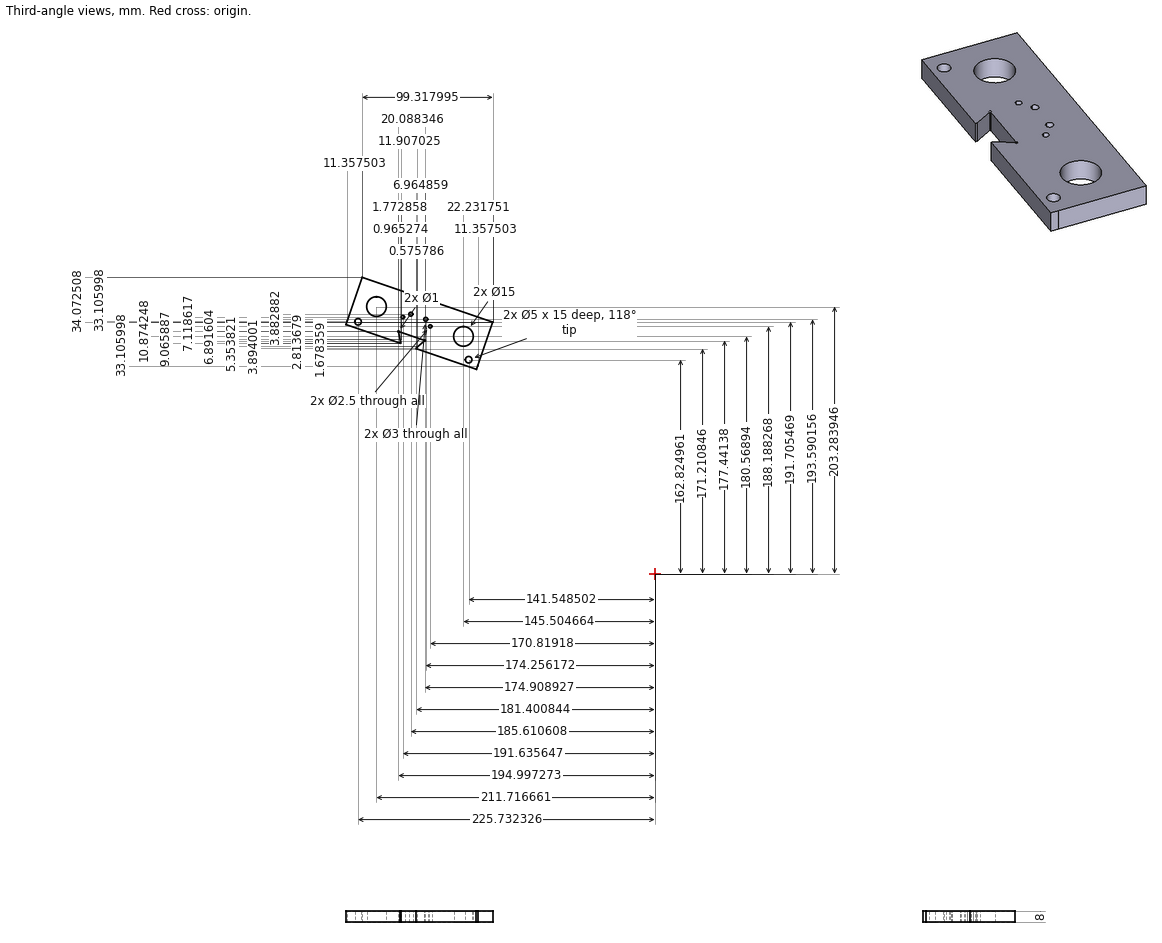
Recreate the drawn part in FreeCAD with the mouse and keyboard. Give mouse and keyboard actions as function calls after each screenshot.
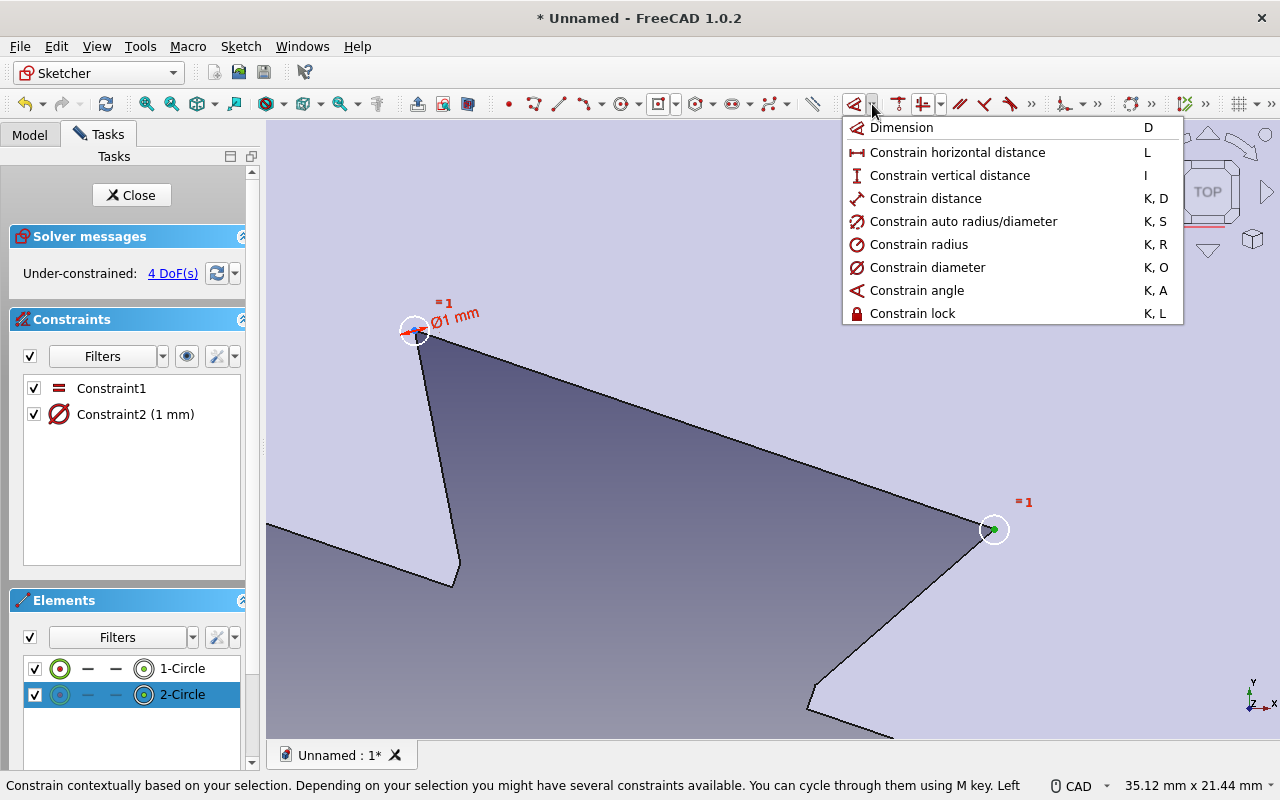
click(1013, 176)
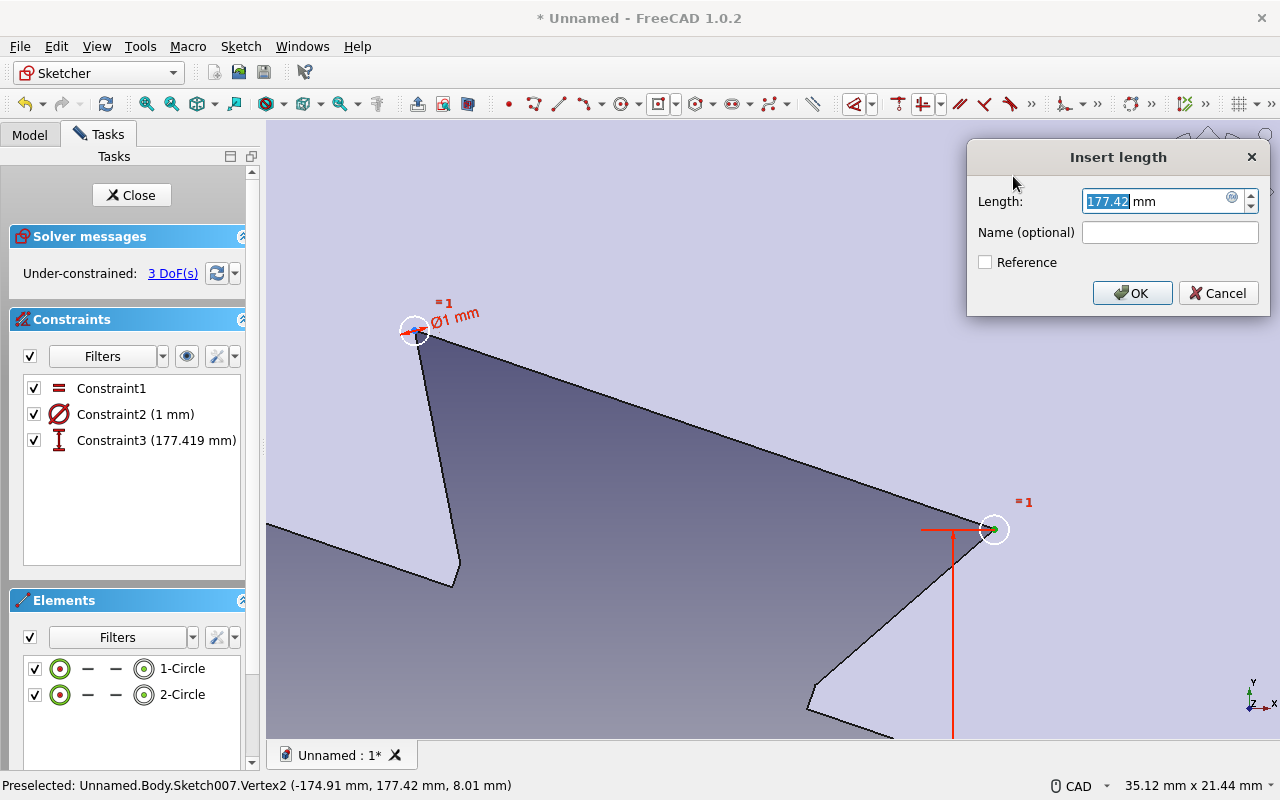
text(177.44138)
key(Return)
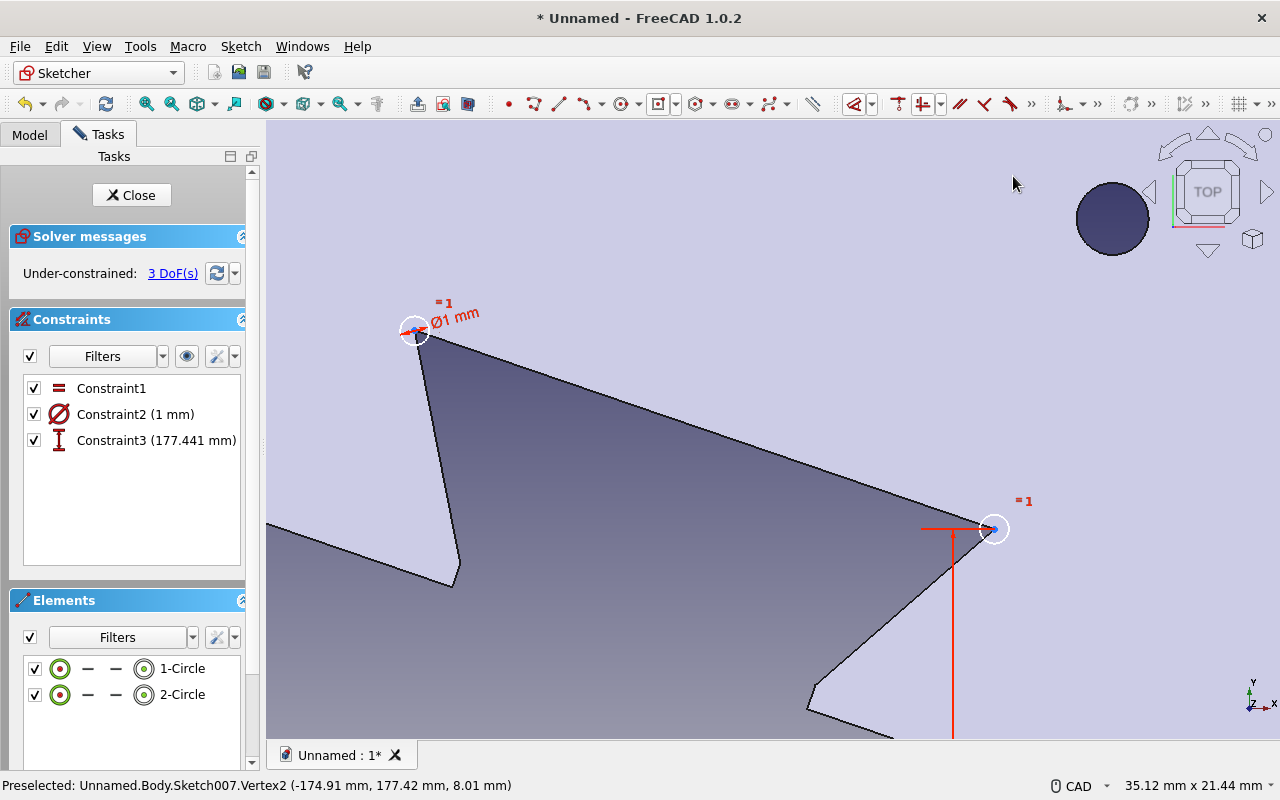
click(415, 331)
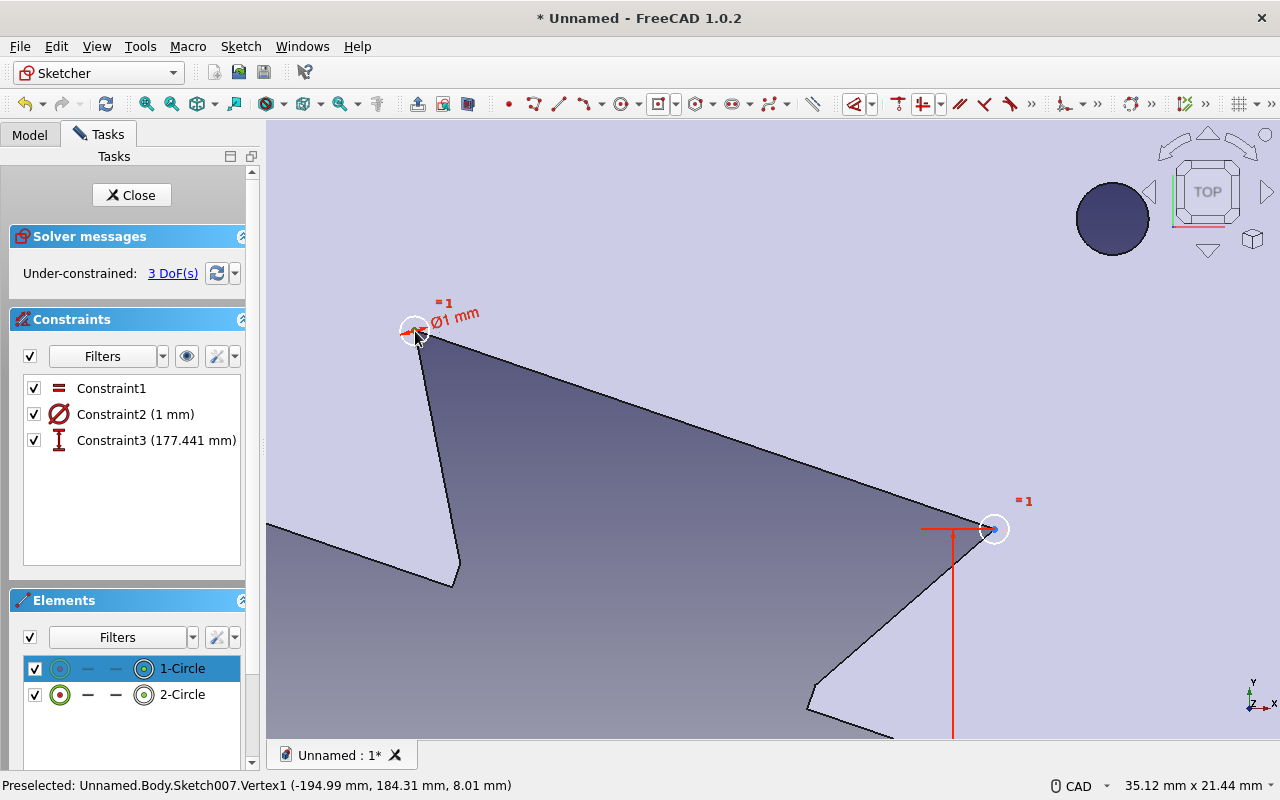
click(994, 529)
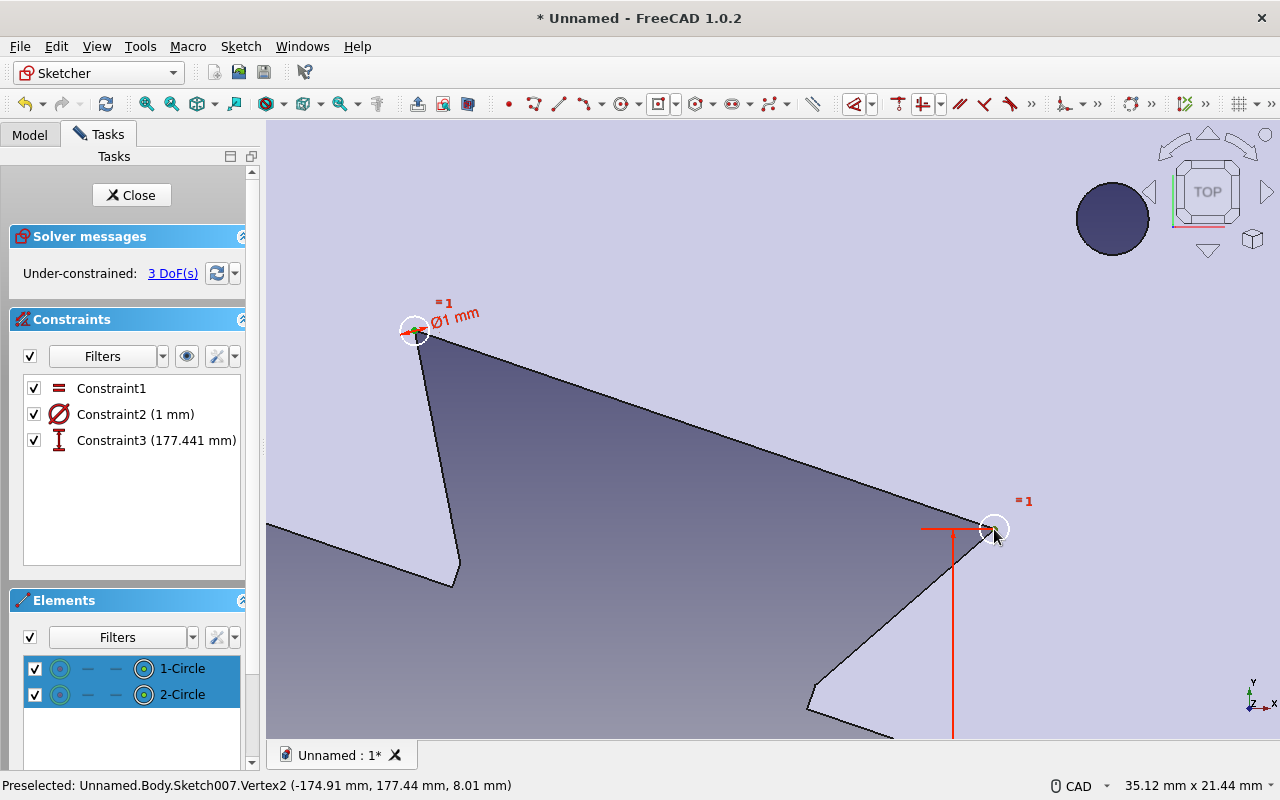
click(872, 104)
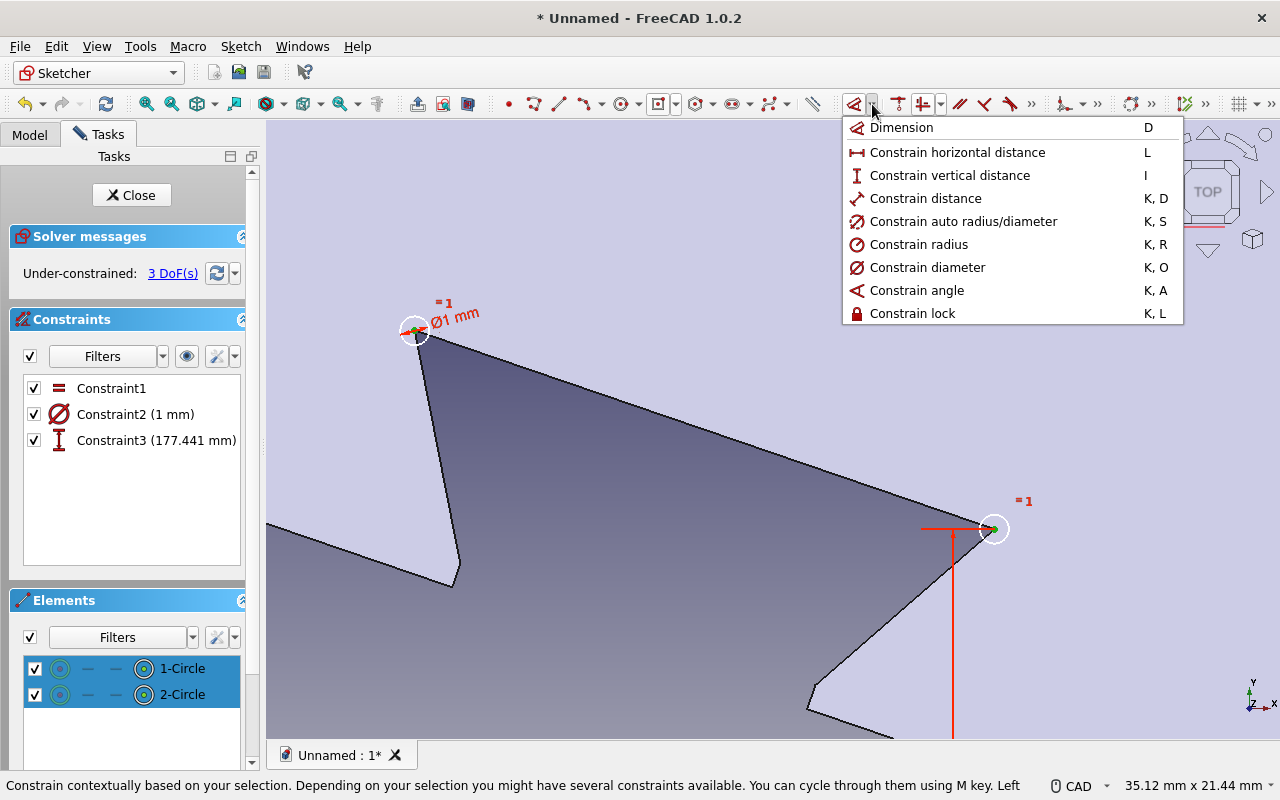
click(1013, 176)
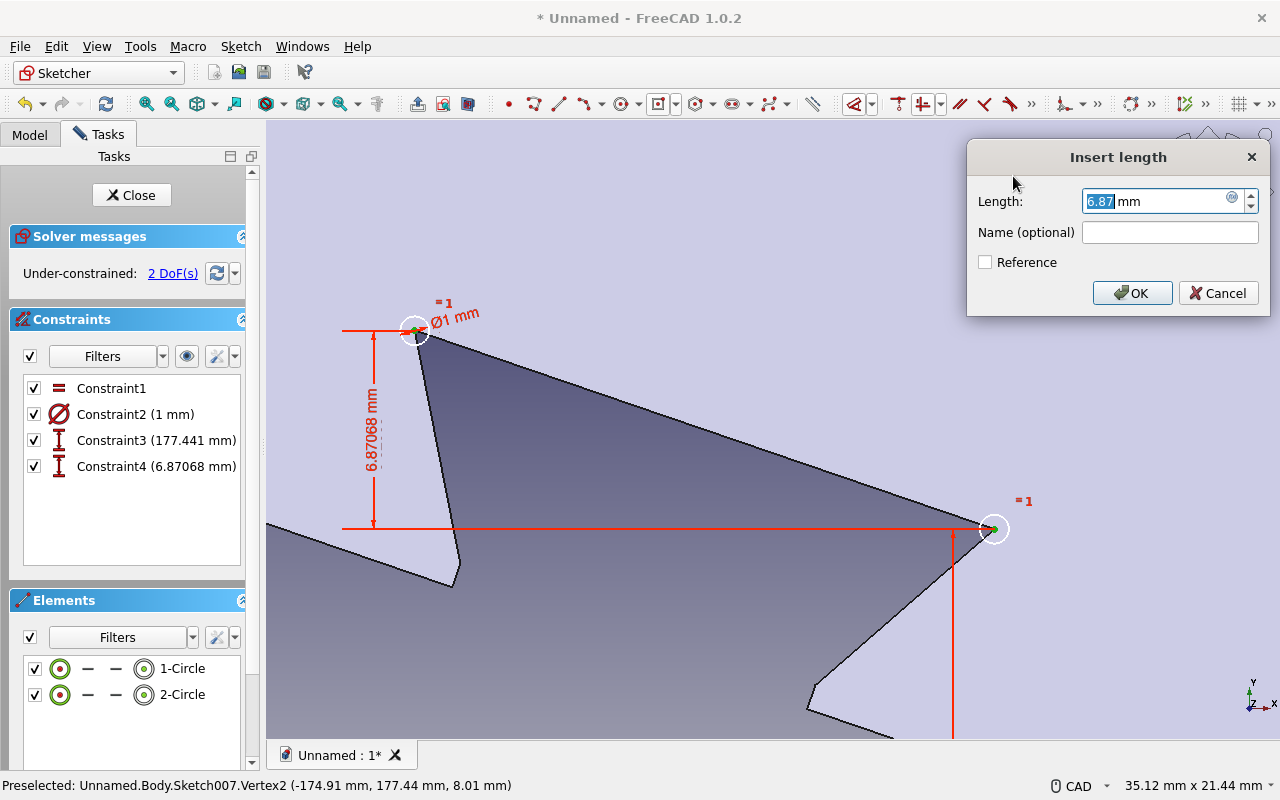
text(6.891604)
key(Return)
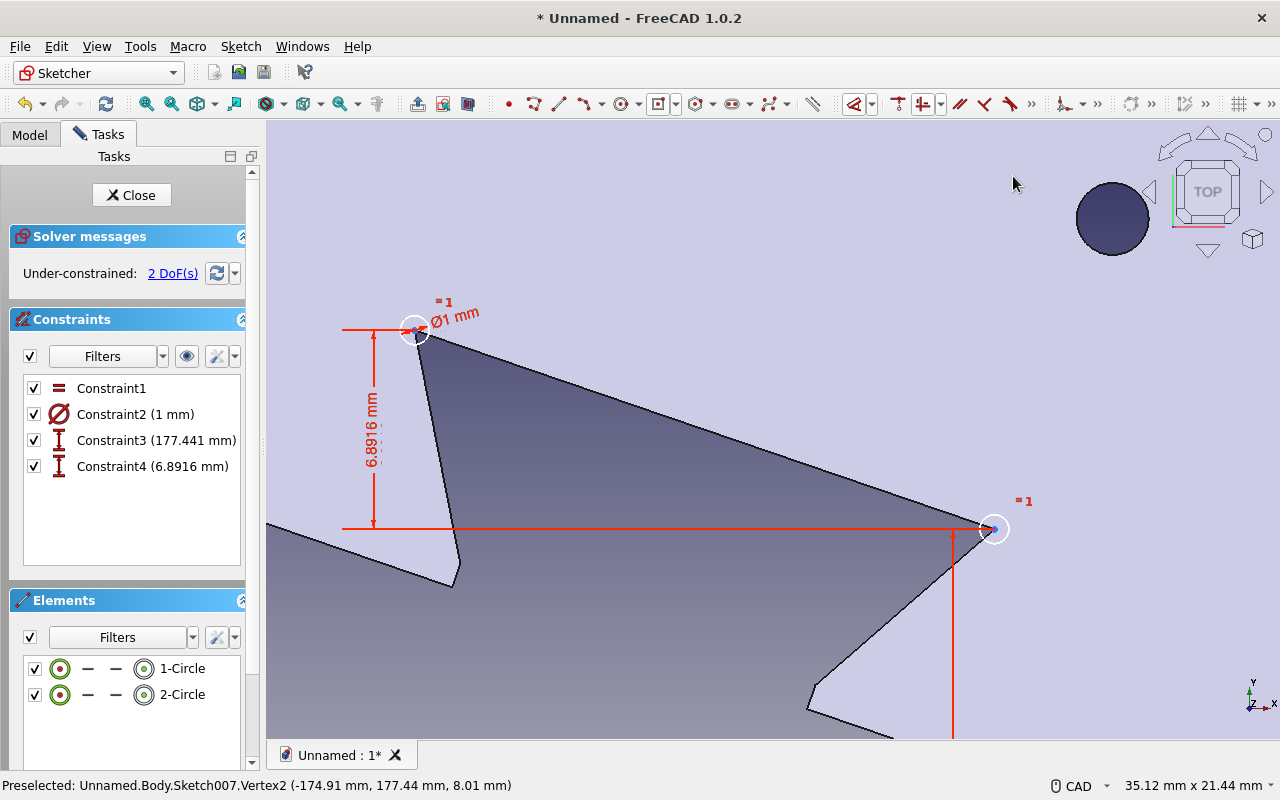
click(415, 330)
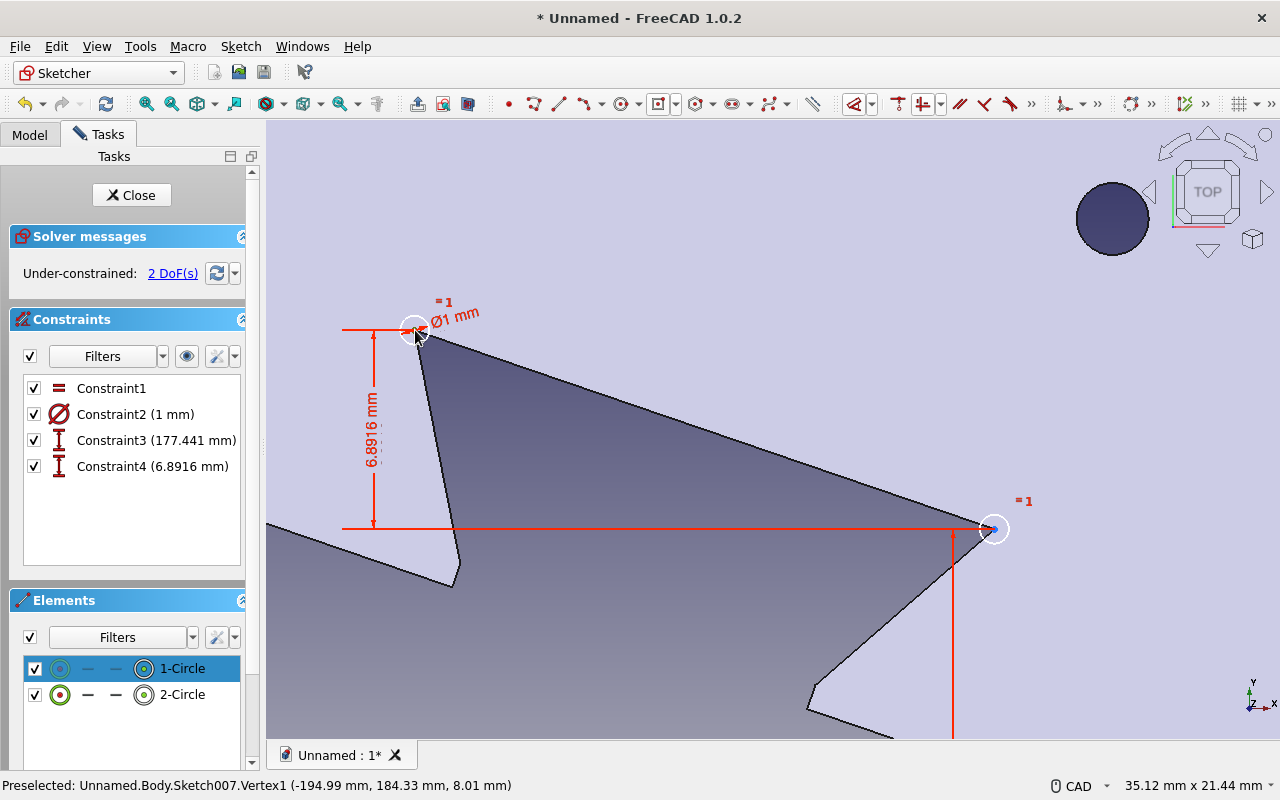
key(l)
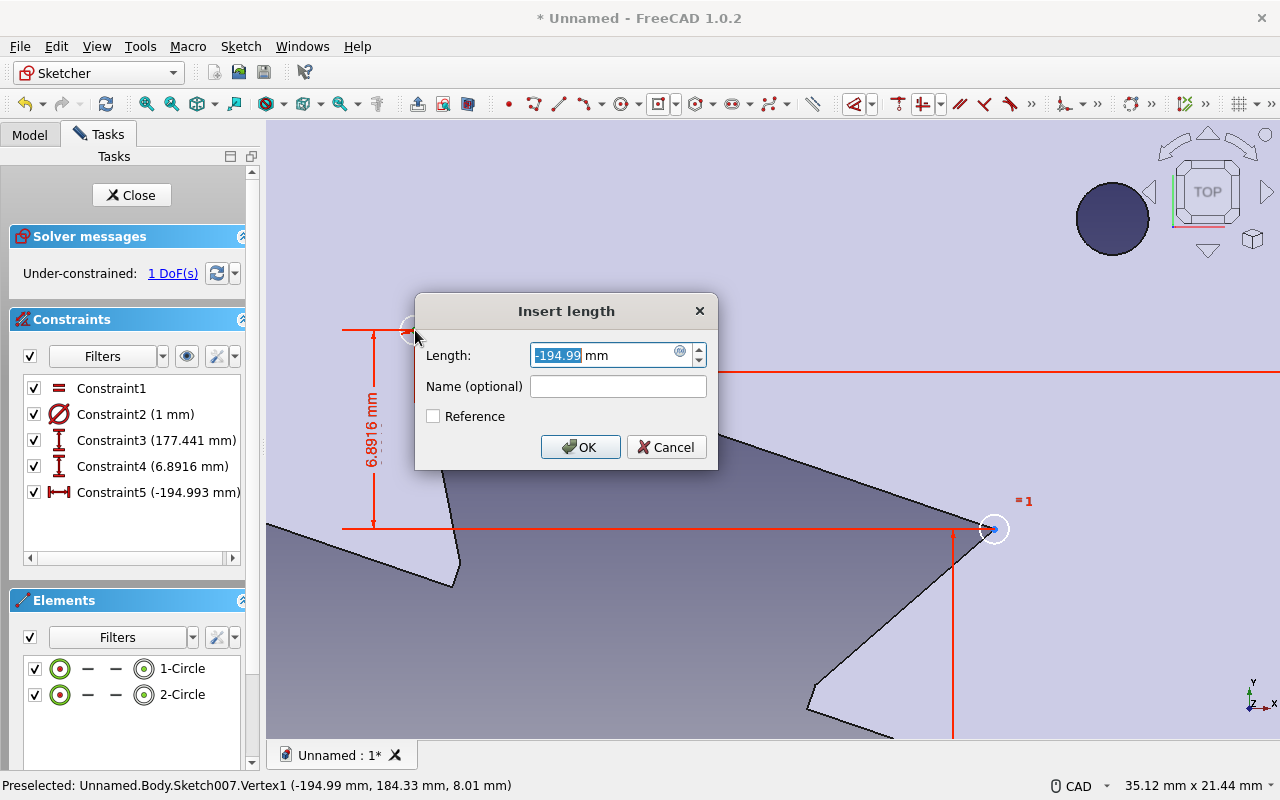
text(-194.997273)
key(Return)